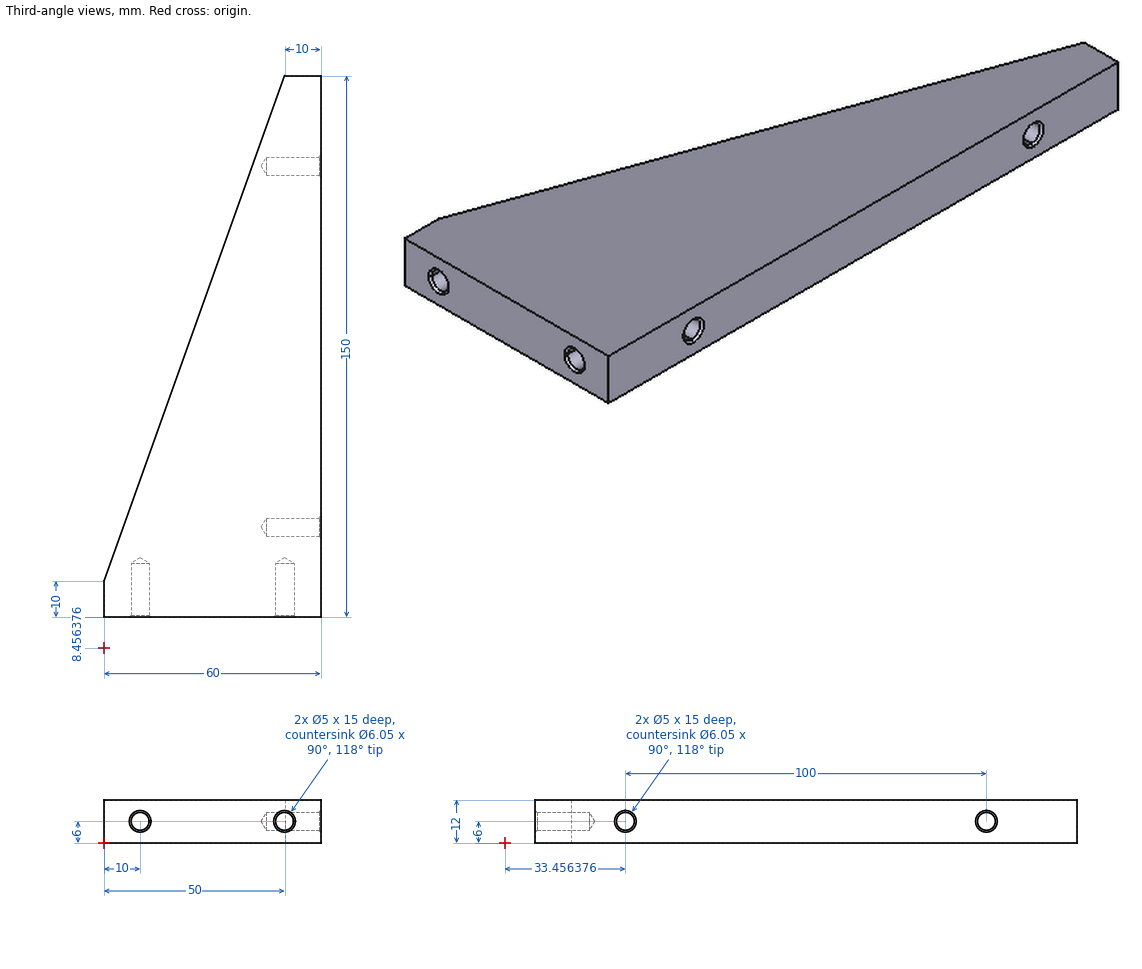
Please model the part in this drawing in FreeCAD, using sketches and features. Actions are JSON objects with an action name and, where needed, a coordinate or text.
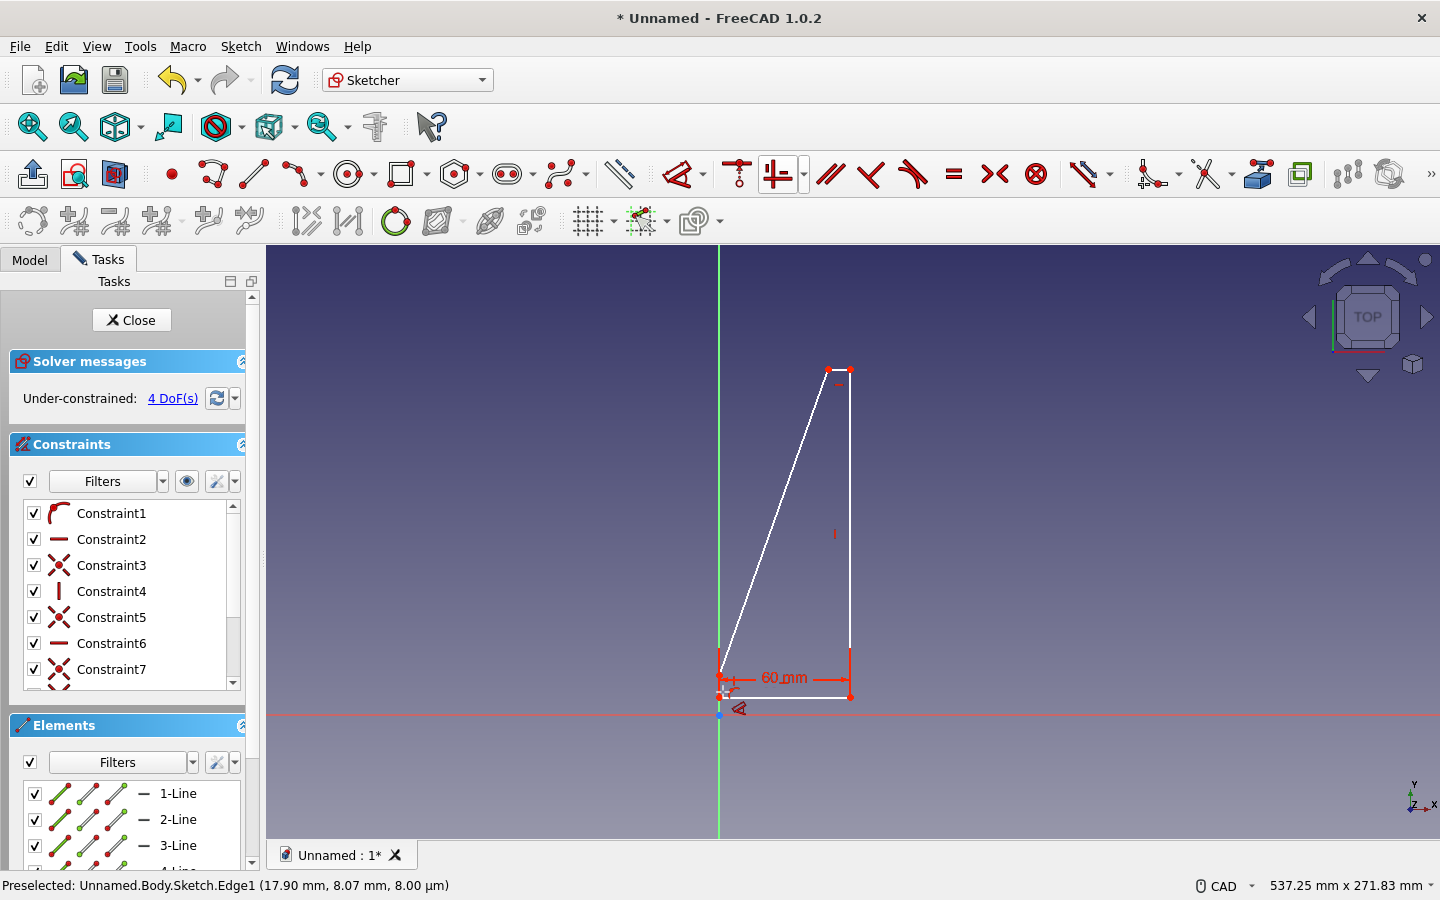
{"action": "scroll", "coordinate": [844, 370], "scroll_direction": "up", "scroll_amount": 4}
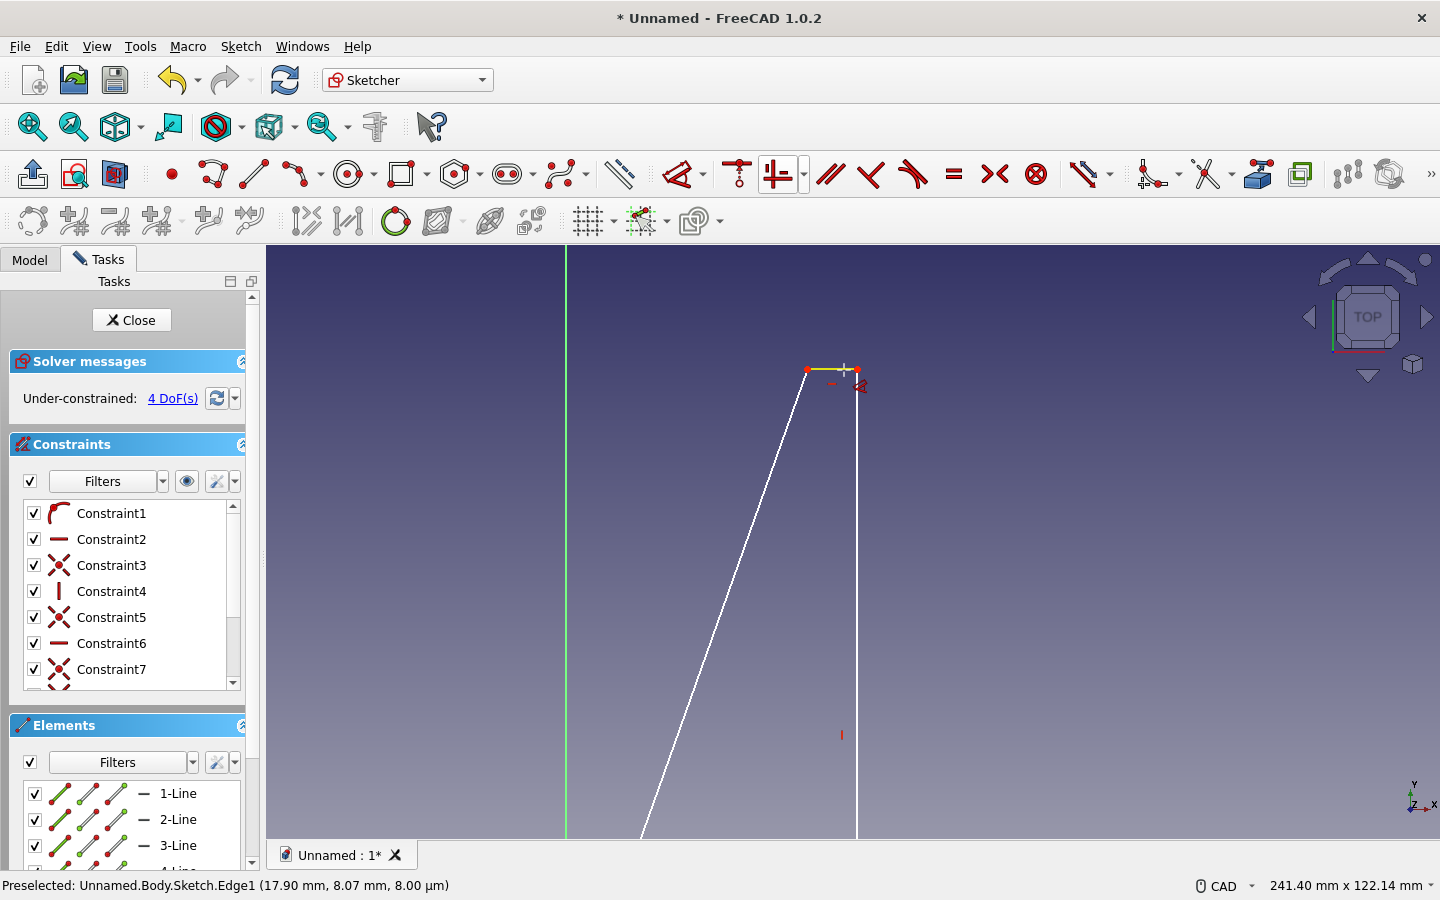
{"action": "left_click", "coordinate": [843, 369]}
{"action": "left_click", "coordinate": [833, 335]}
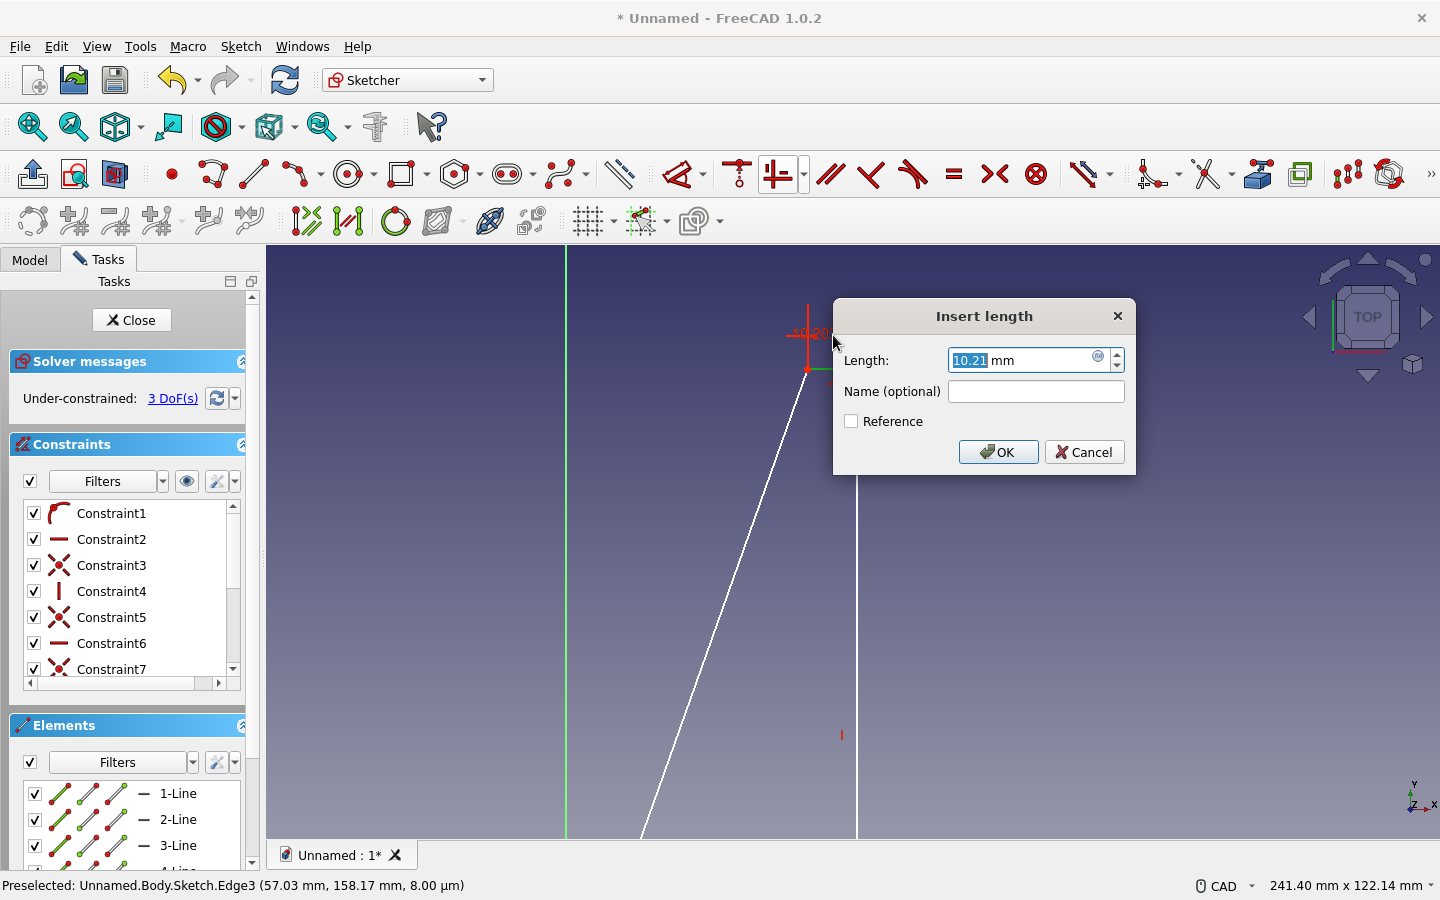
{"action": "type", "text": "10"}
{"action": "key", "text": "Return"}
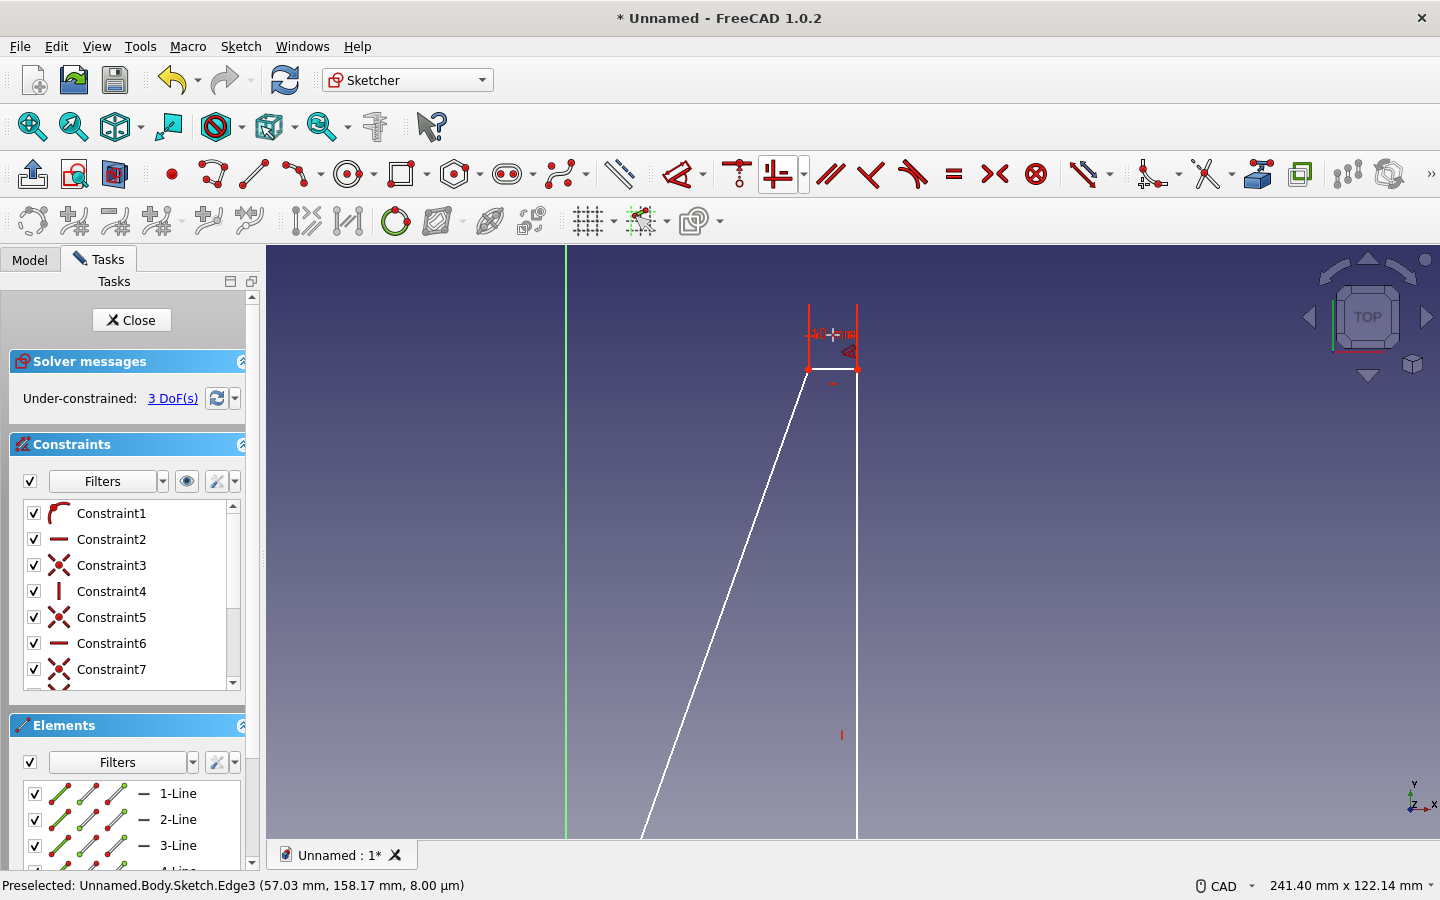
{"action": "scroll", "coordinate": [844, 370], "scroll_direction": "down", "scroll_amount": 4}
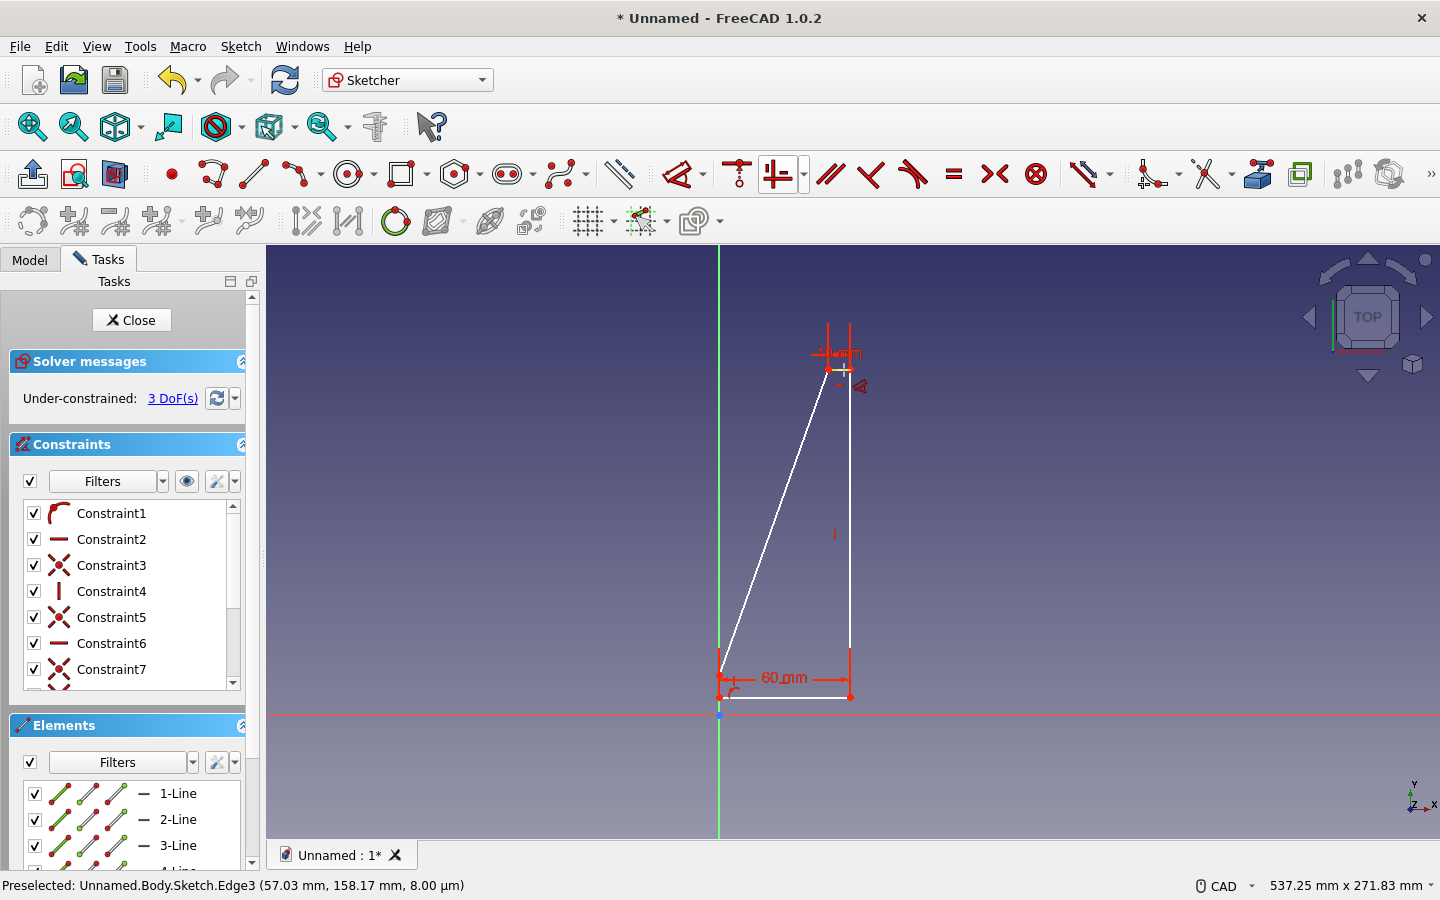
{"action": "scroll", "coordinate": [719, 682], "scroll_direction": "up", "scroll_amount": 4}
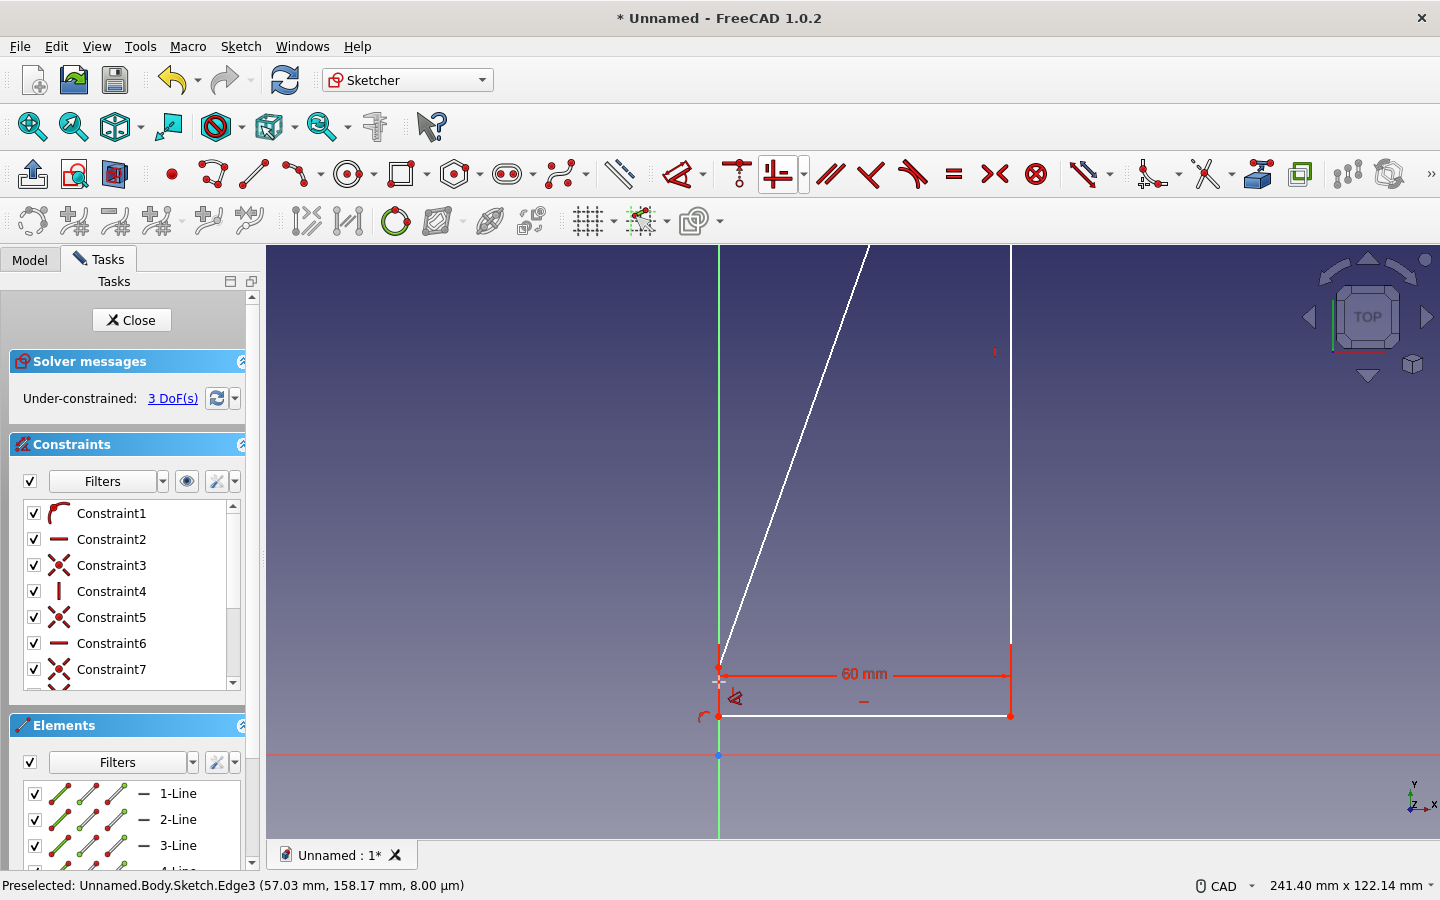
{"action": "left_click", "coordinate": [719, 682]}
{"action": "left_click", "coordinate": [685, 692]}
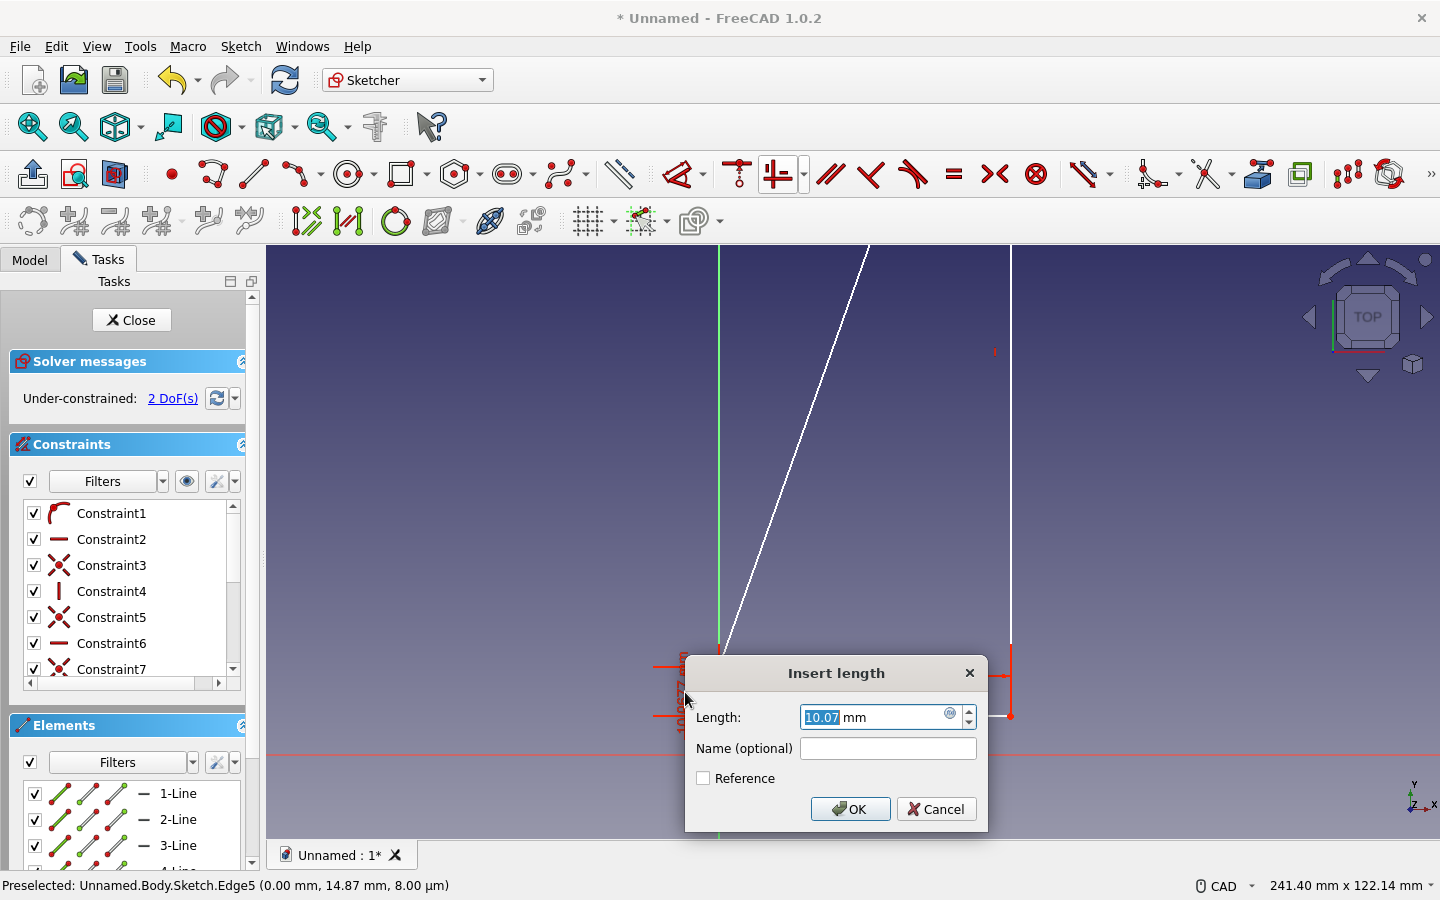
{"action": "type", "text": "10"}
{"action": "key", "text": "Return"}